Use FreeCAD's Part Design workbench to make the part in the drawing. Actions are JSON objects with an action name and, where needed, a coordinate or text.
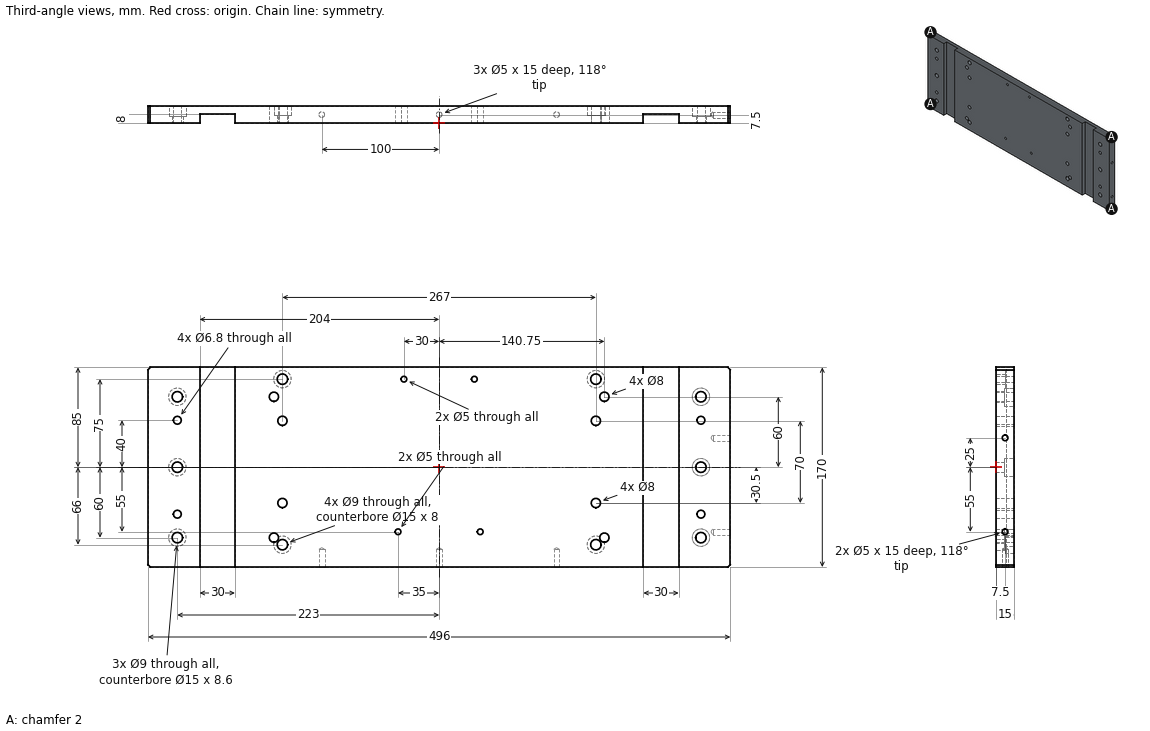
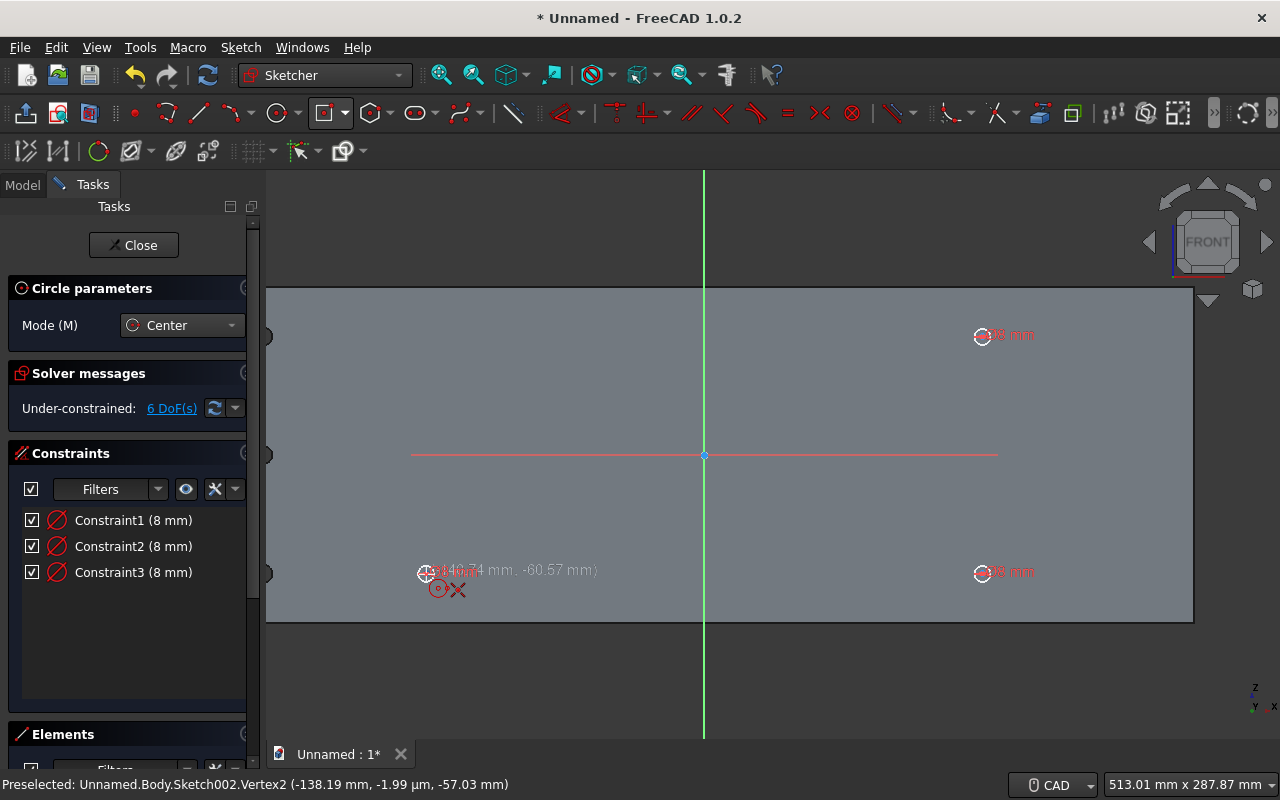
{"action": "scroll", "coordinate": [426, 336], "scroll_direction": "up", "scroll_amount": 6}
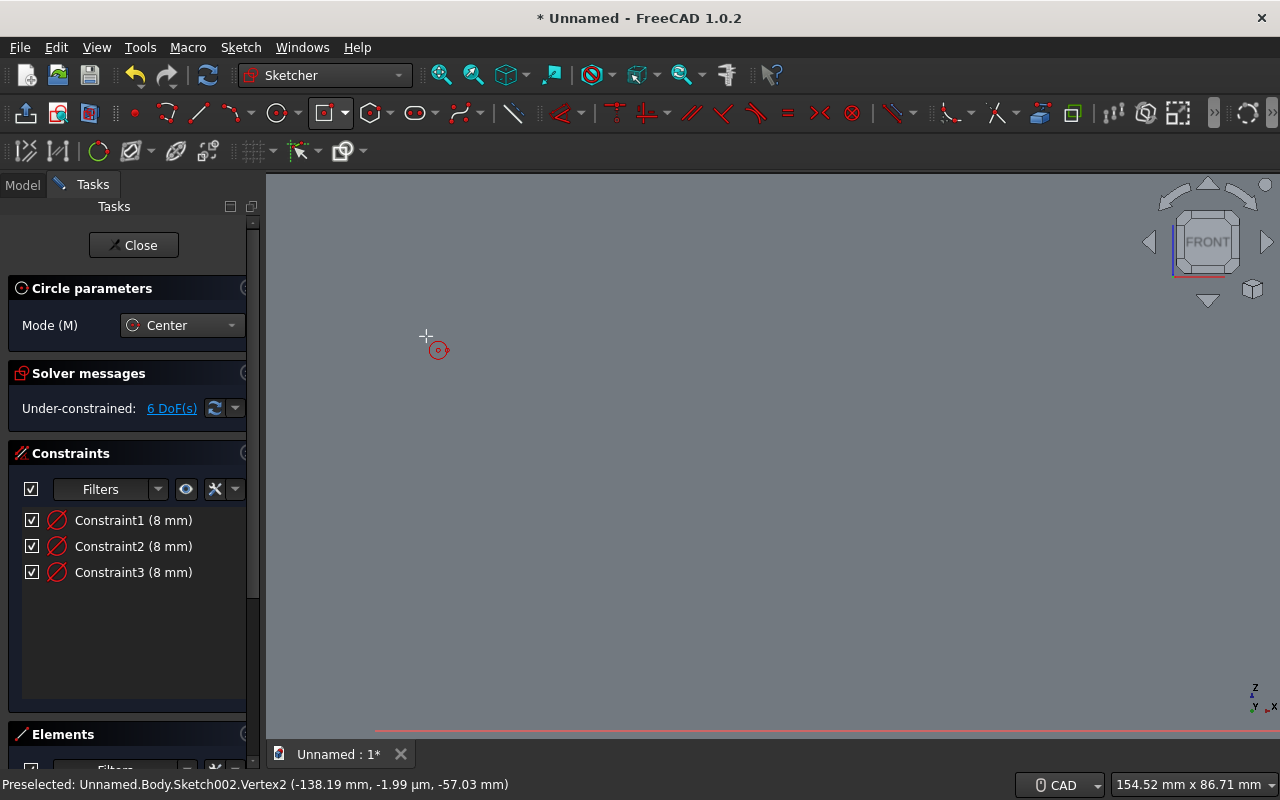
{"action": "left_click", "coordinate": [426, 337]}
{"action": "mouse_move", "coordinate": [444, 318]}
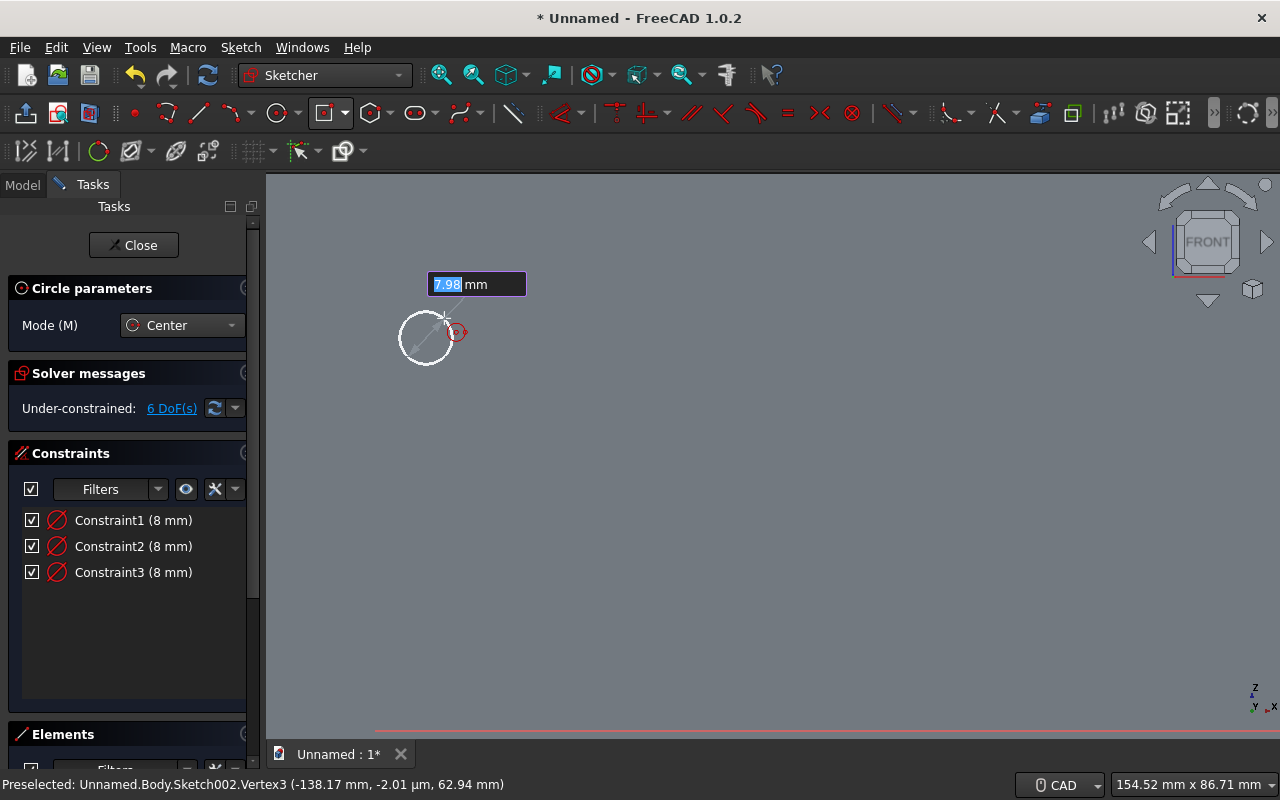
{"action": "type", "text": "8"}
{"action": "key", "text": "Return"}
{"action": "key", "text": "Escape"}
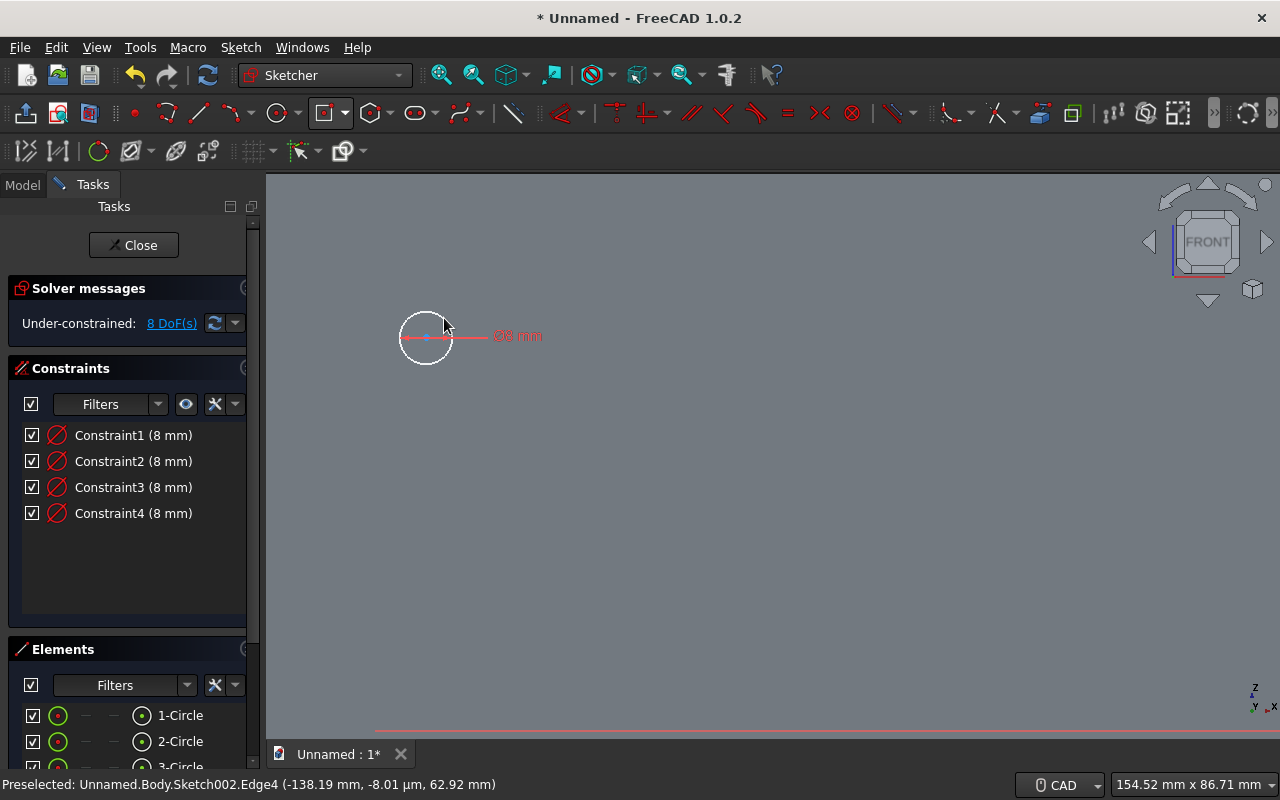
{"action": "scroll", "coordinate": [426, 335], "scroll_direction": "down", "scroll_amount": 6}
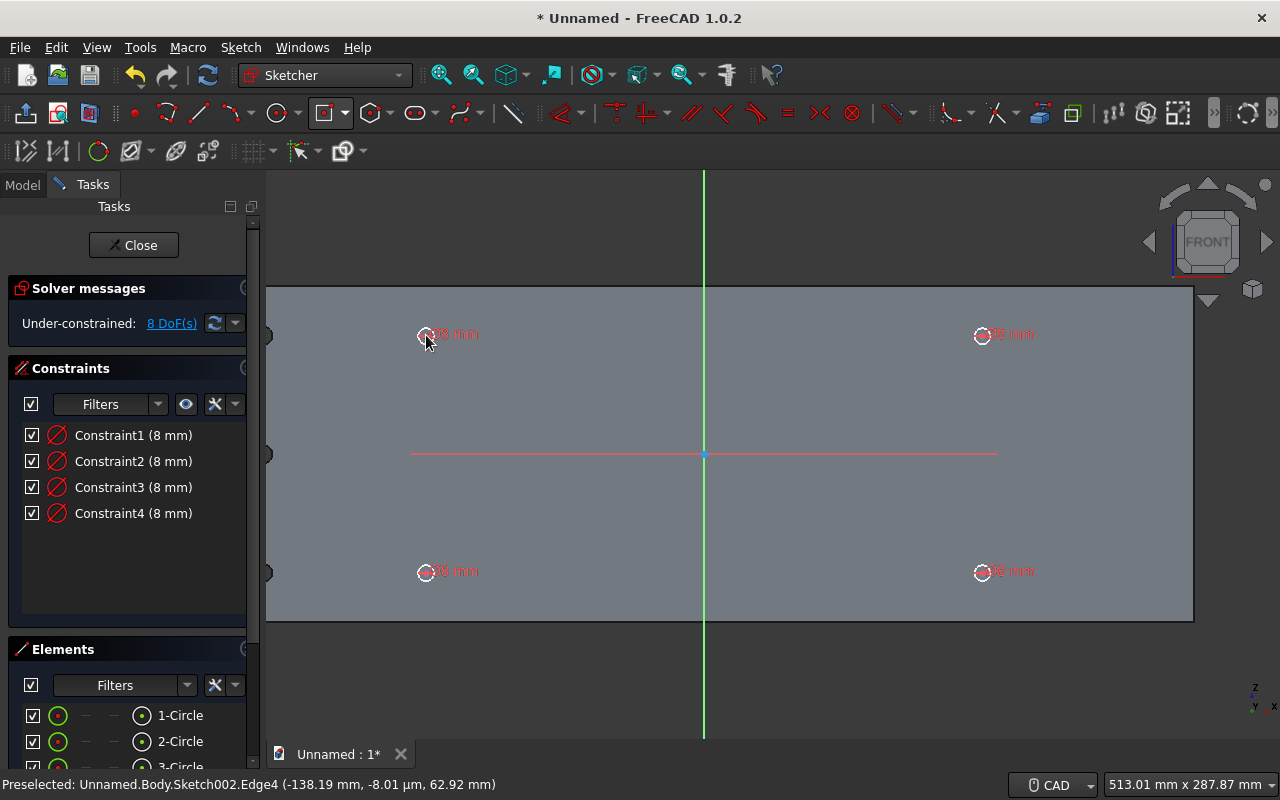
{"action": "left_click", "coordinate": [982, 336]}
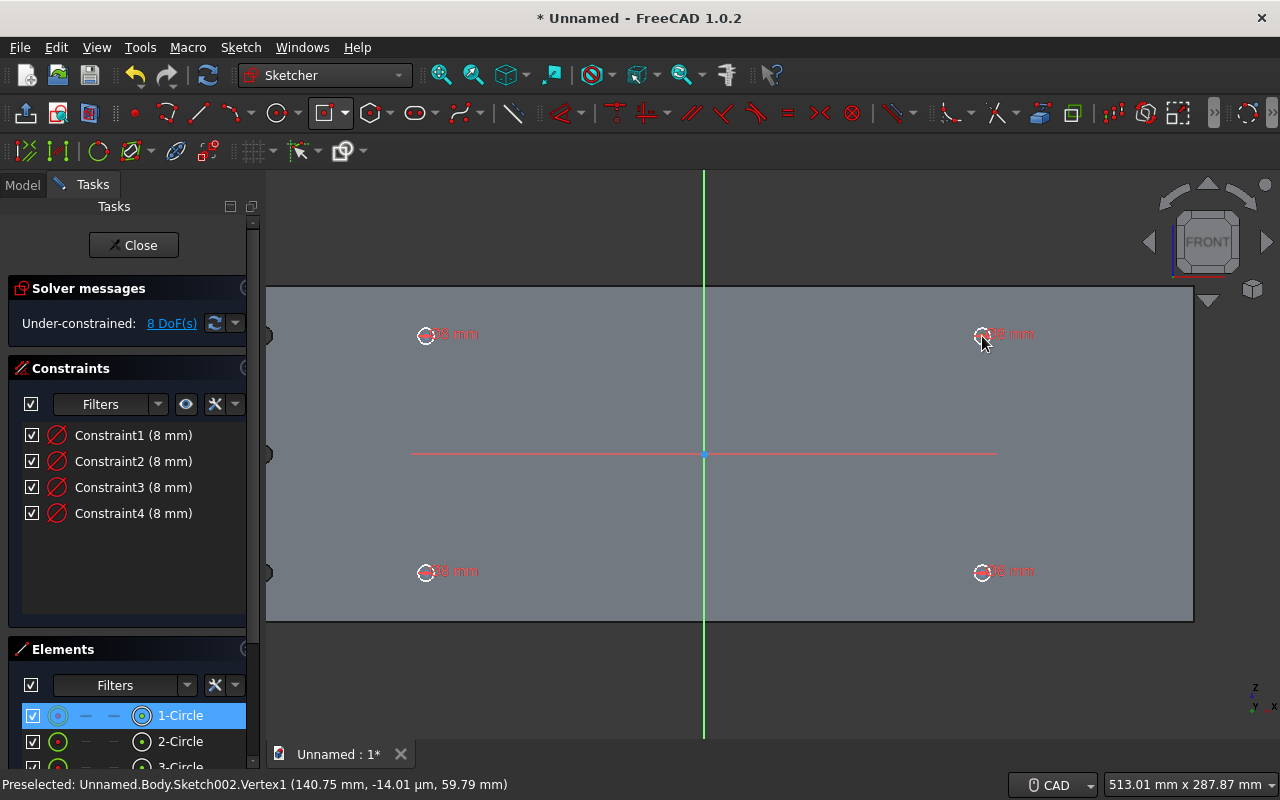
{"action": "left_click", "coordinate": [982, 573]}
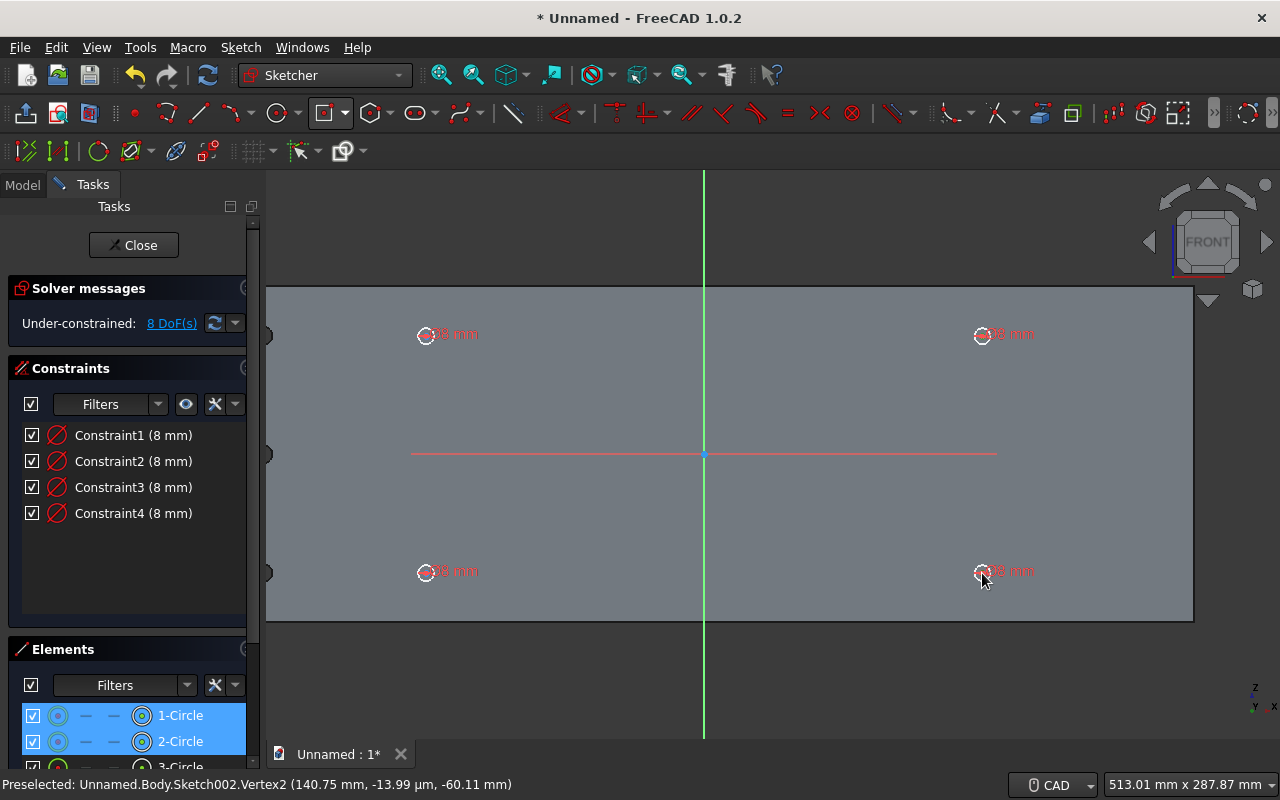
{"action": "left_click", "coordinate": [411, 454]}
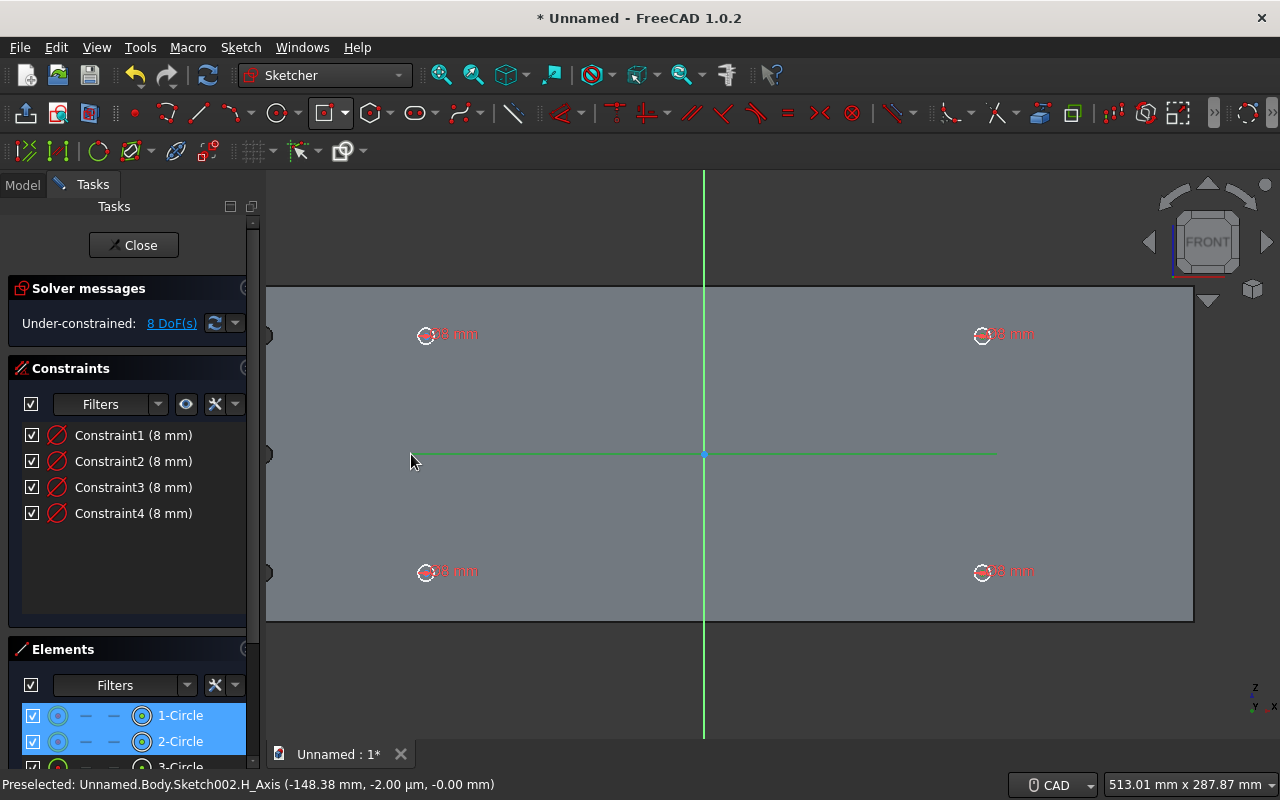
{"action": "left_click", "coordinate": [820, 114]}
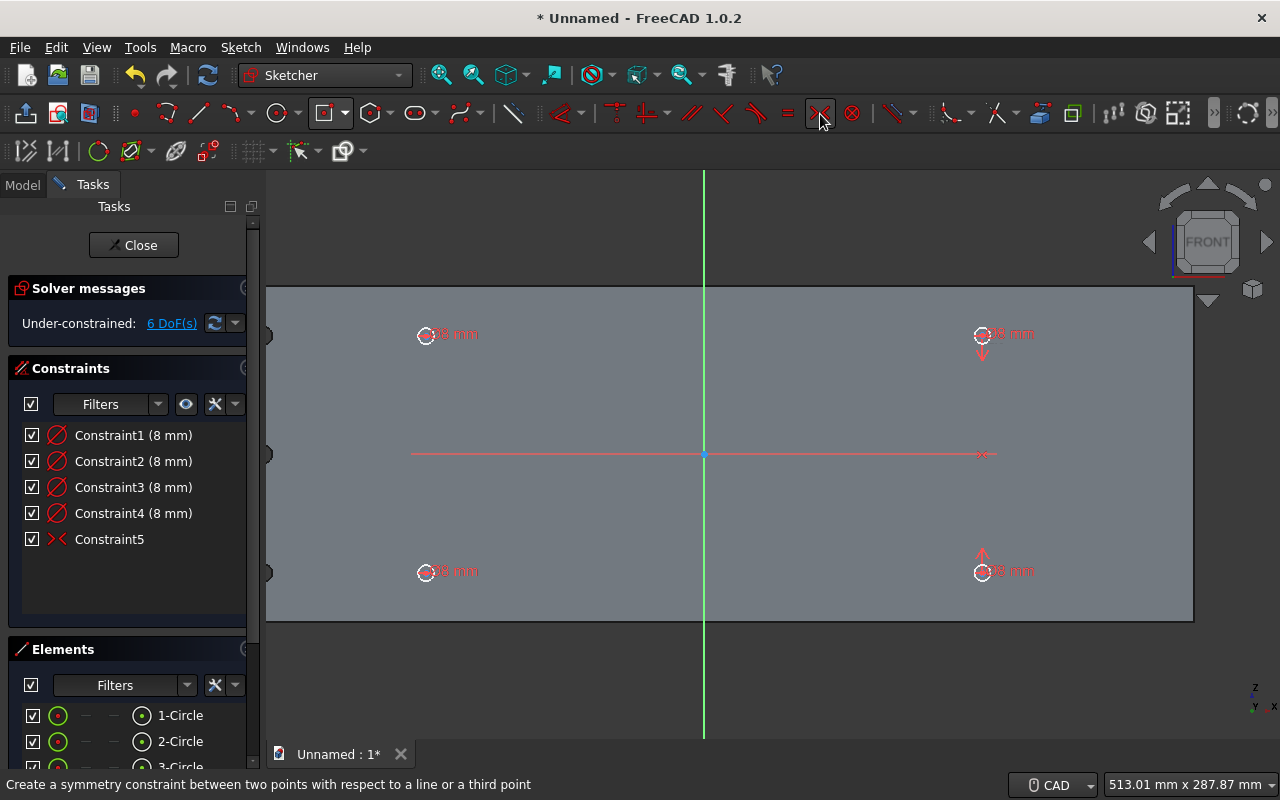
{"action": "left_click", "coordinate": [982, 573]}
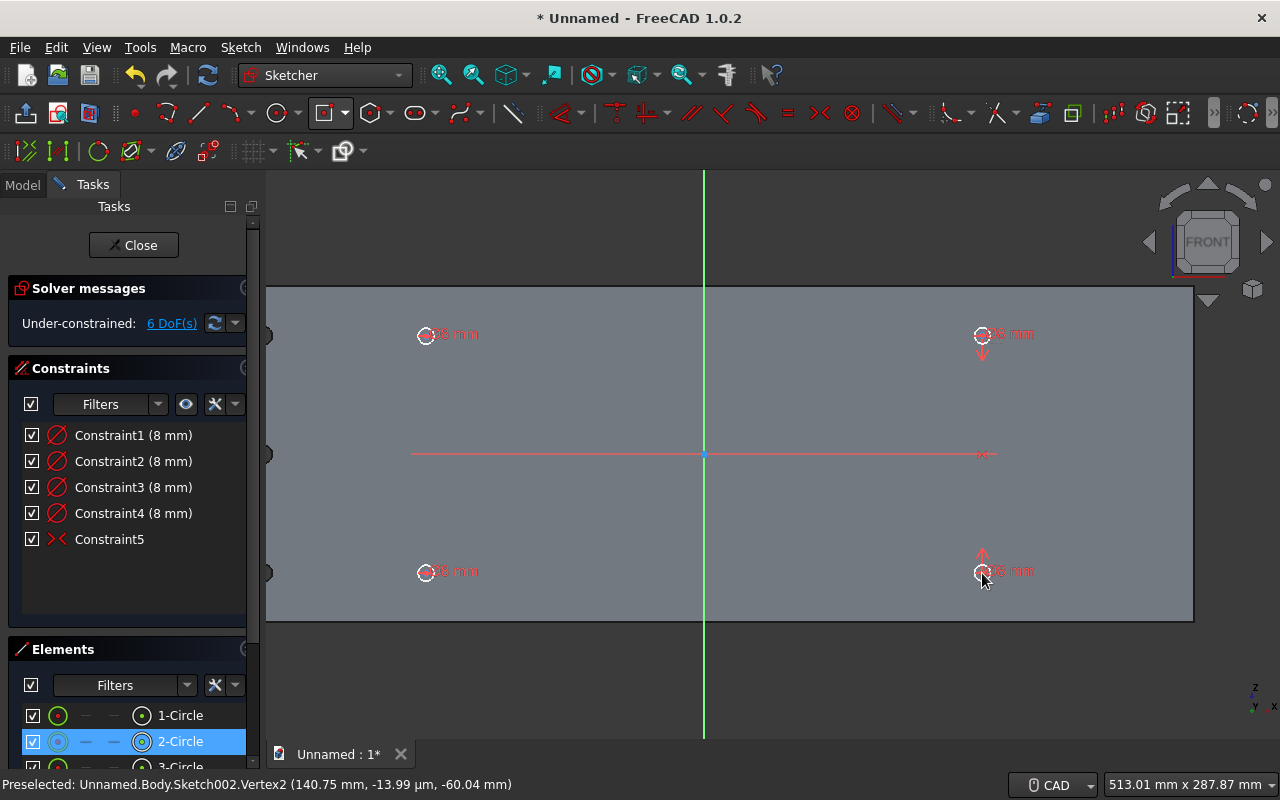
{"action": "left_click", "coordinate": [426, 573]}